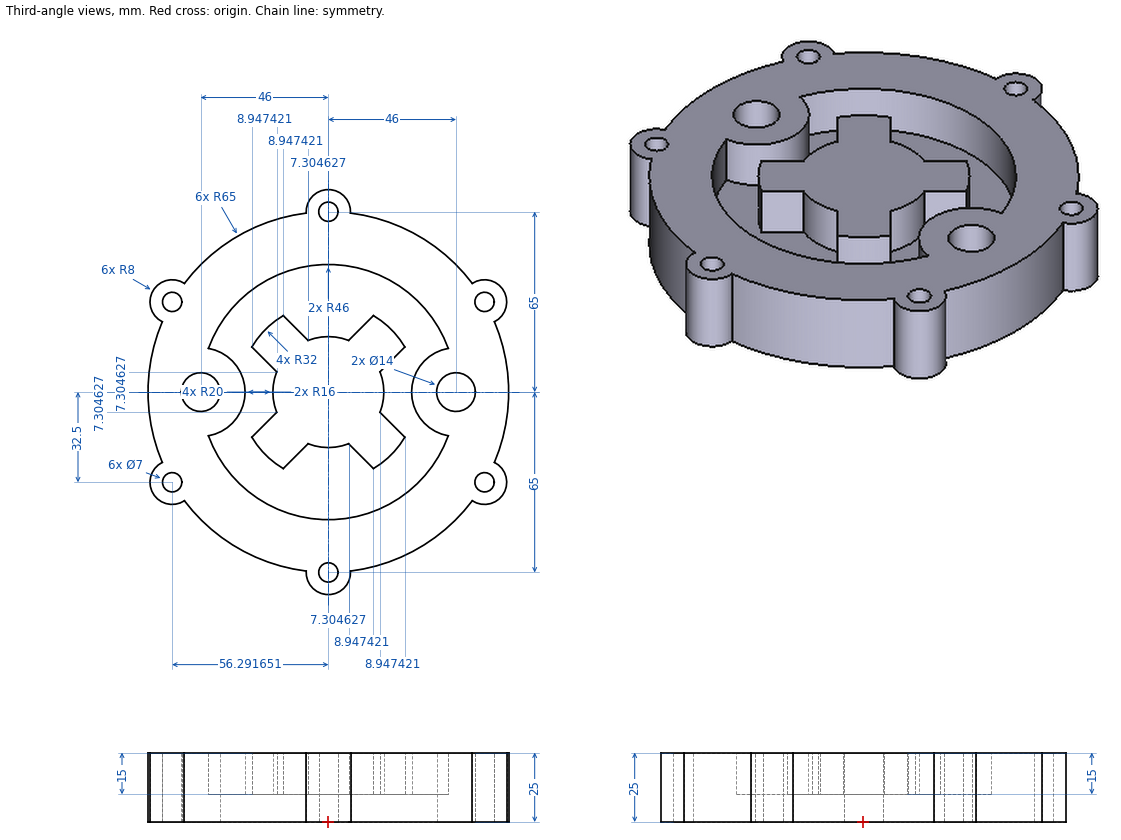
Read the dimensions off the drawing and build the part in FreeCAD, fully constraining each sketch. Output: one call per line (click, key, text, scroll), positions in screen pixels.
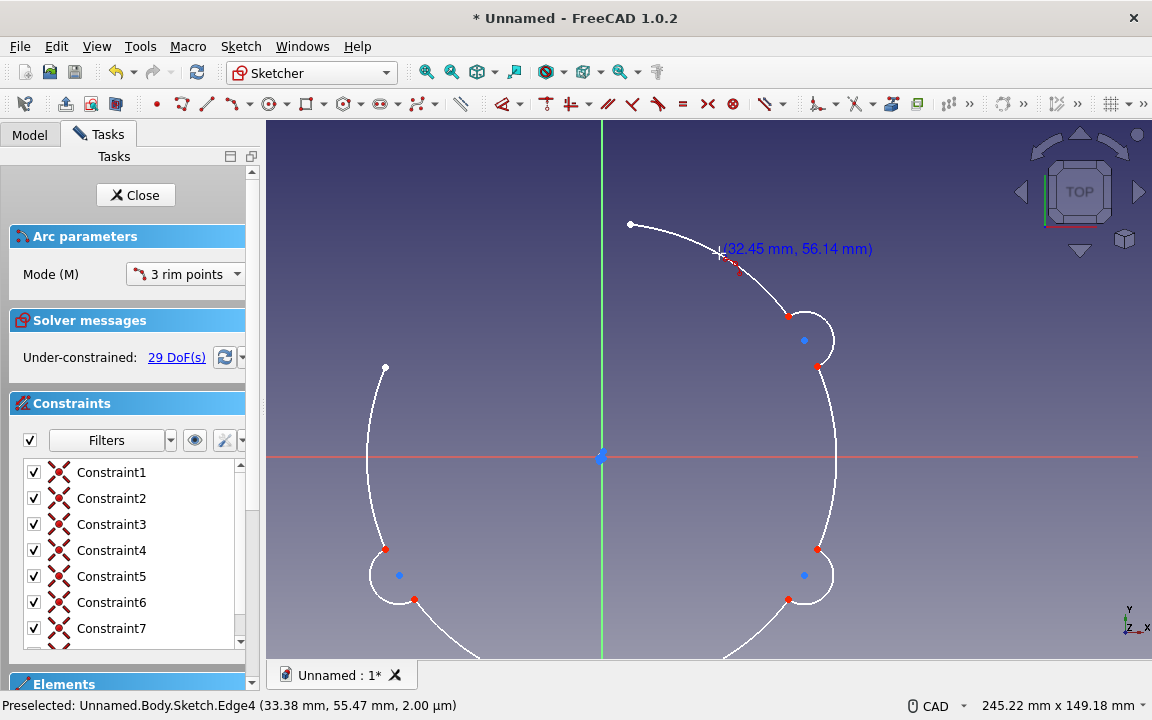
click(631, 225)
click(573, 224)
click(619, 199)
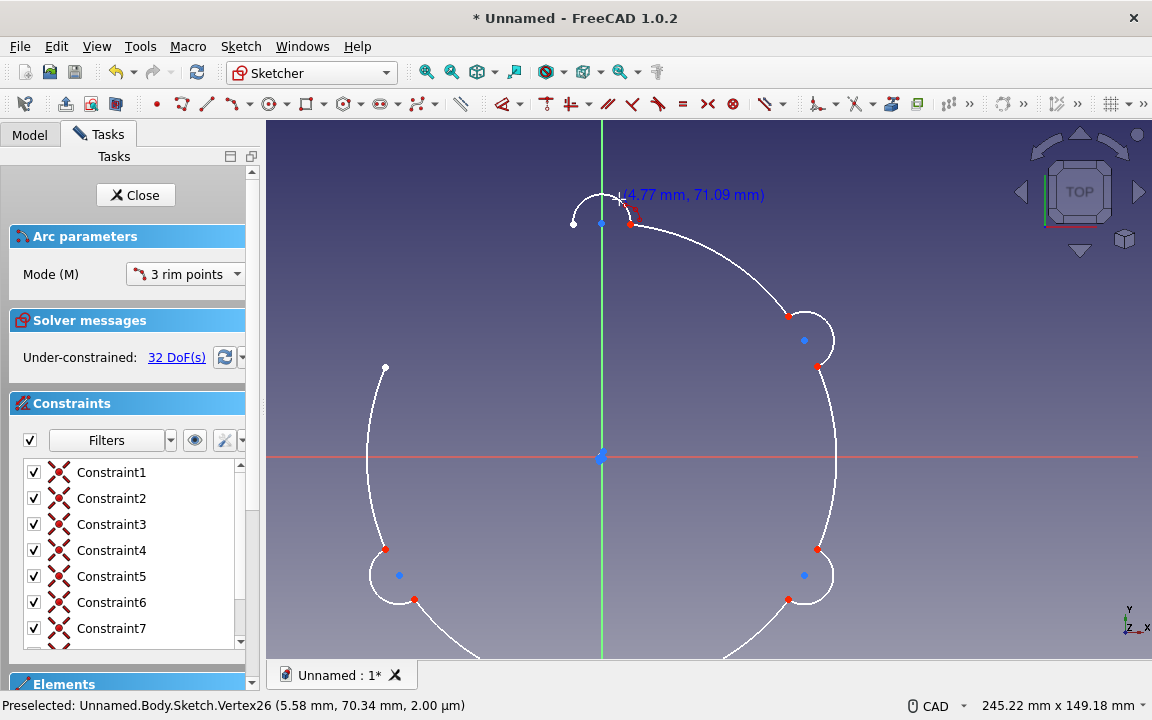
click(573, 225)
click(414, 315)
click(484, 253)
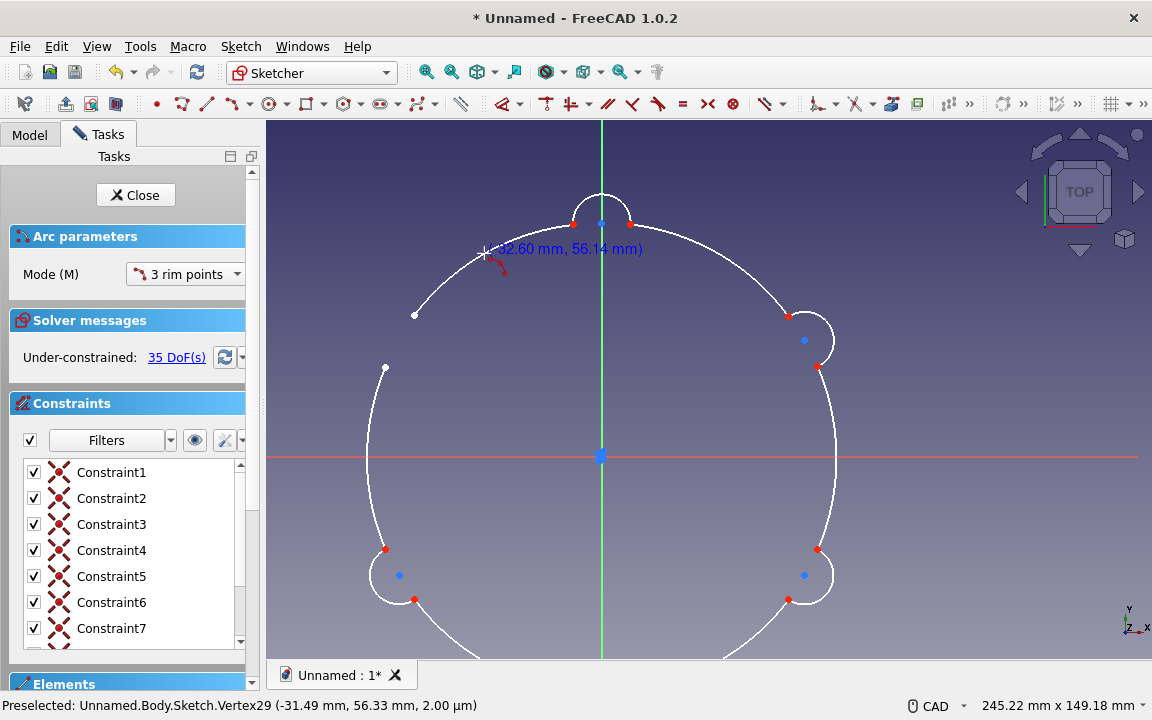
click(414, 316)
click(386, 367)
click(373, 325)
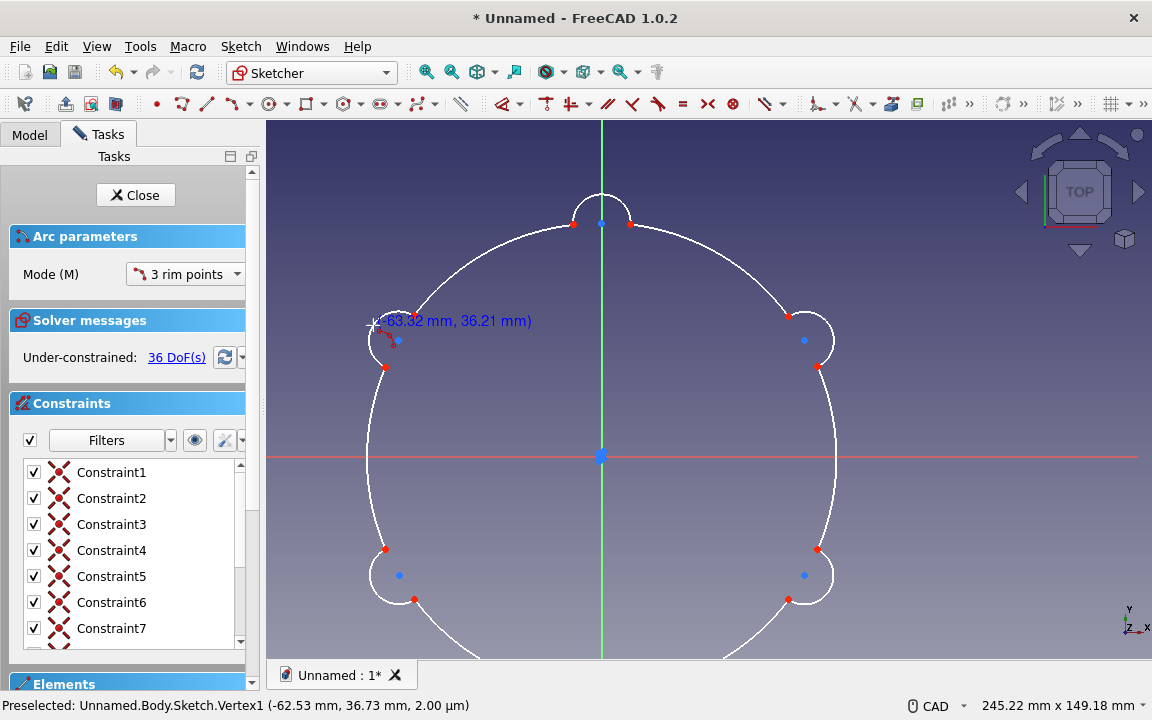
click(268, 104)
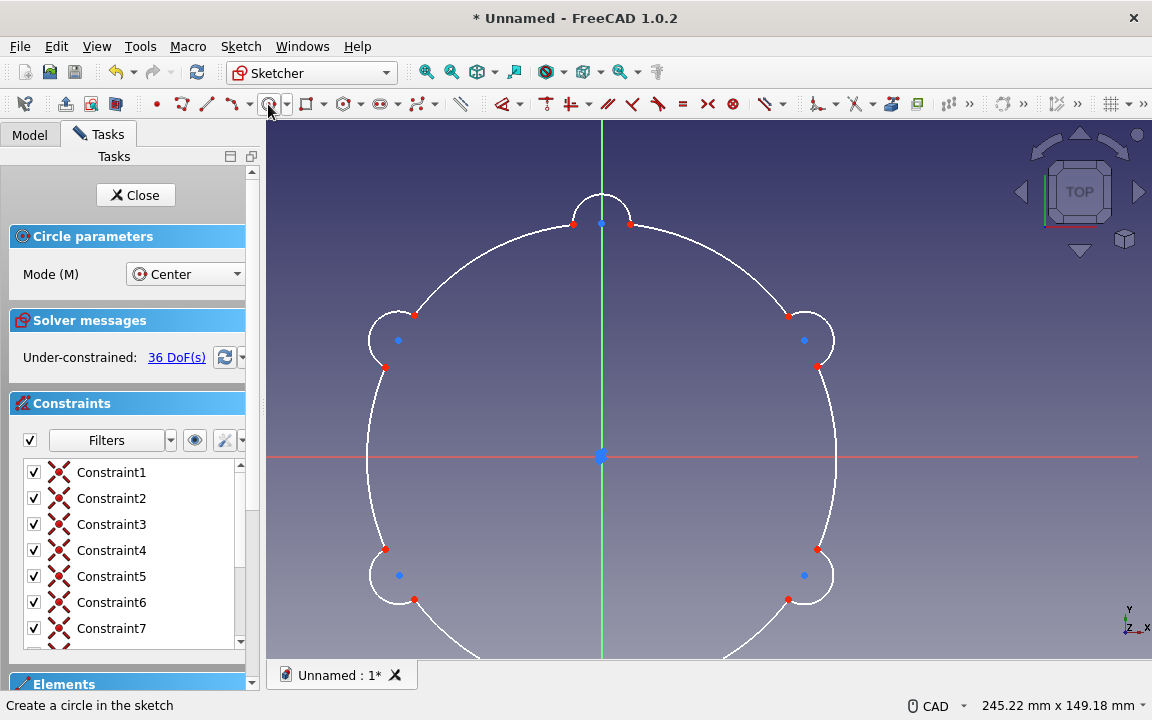
scroll(398, 574, up, 3)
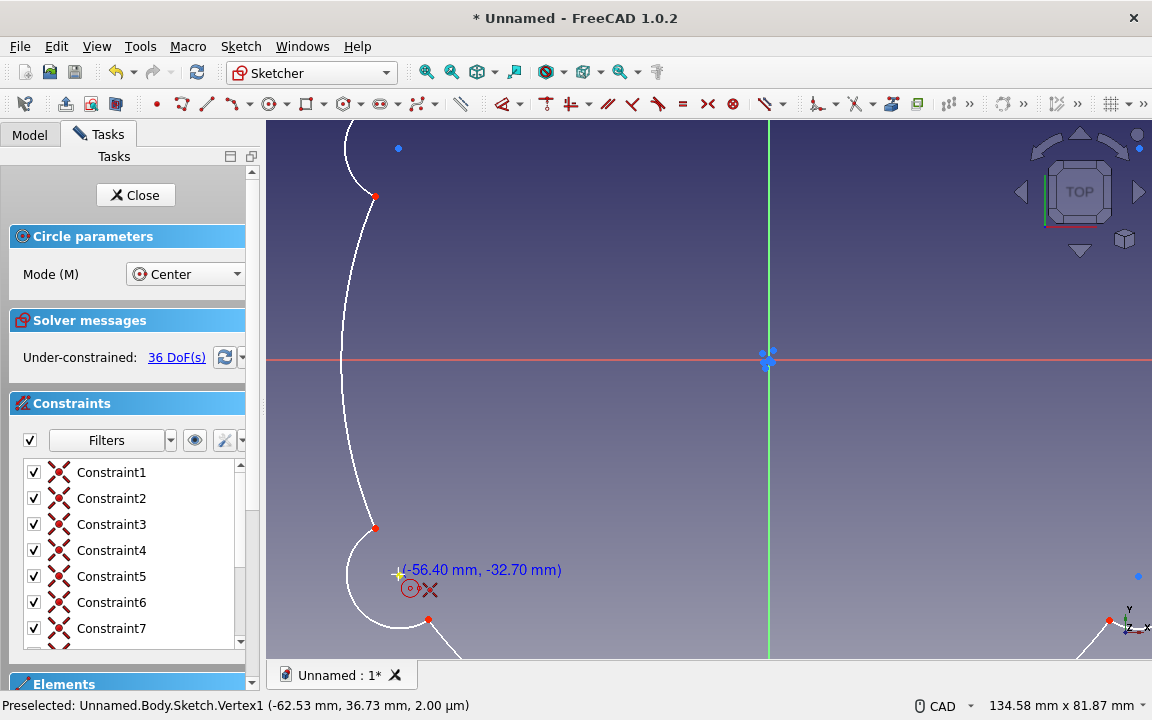
click(399, 574)
click(415, 557)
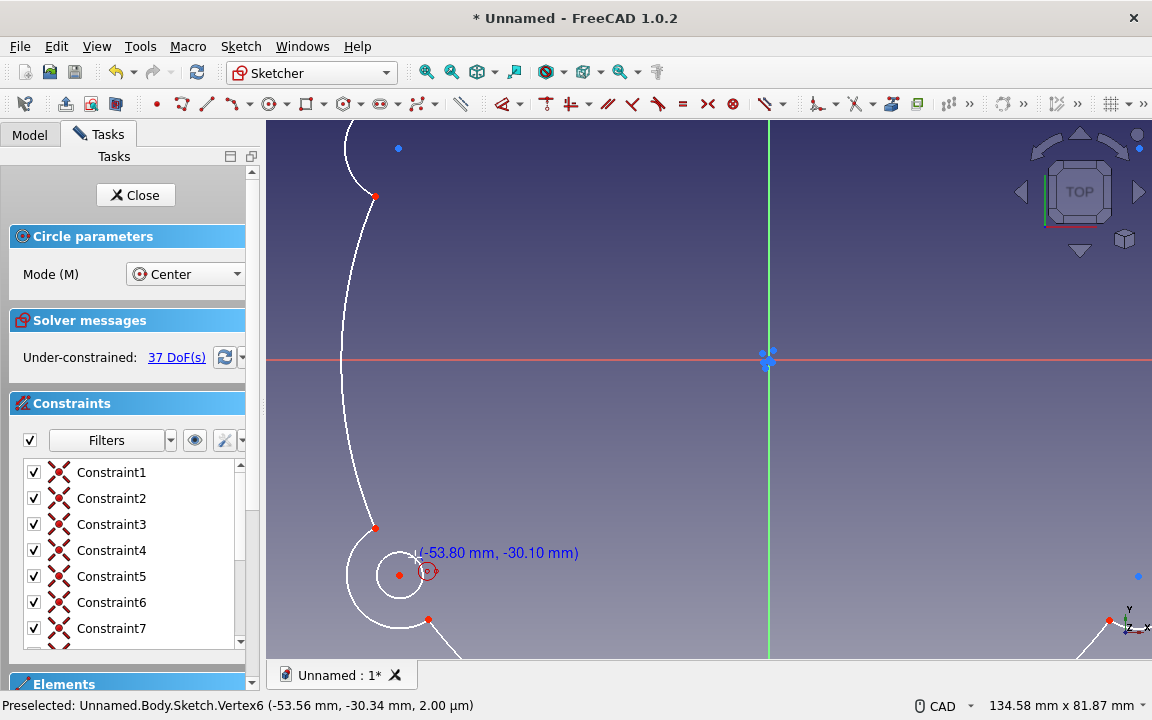
scroll(566, 407, down, 5)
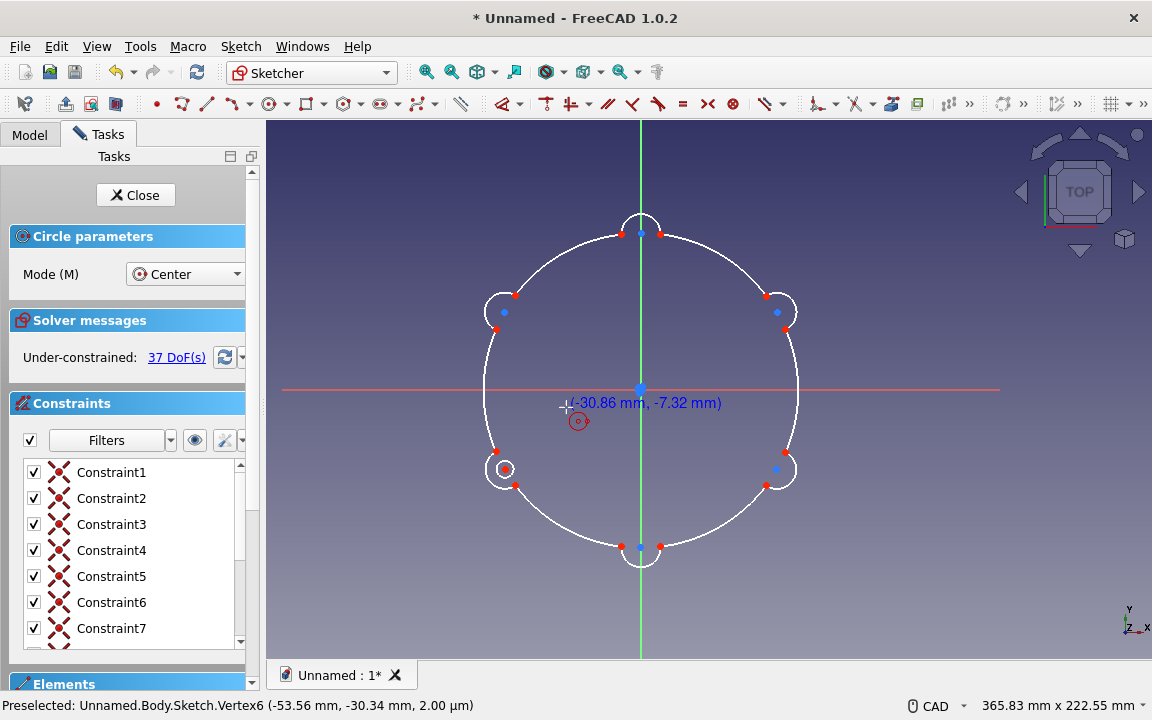
scroll(641, 547, up, 5)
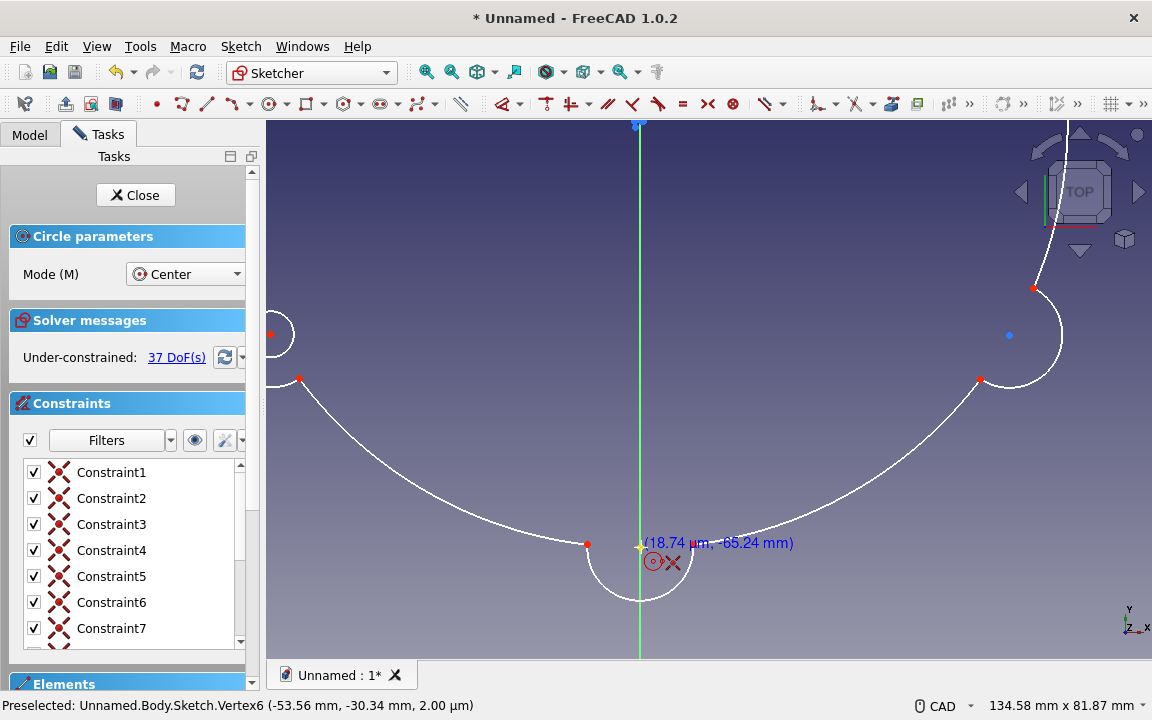
click(640, 547)
click(656, 530)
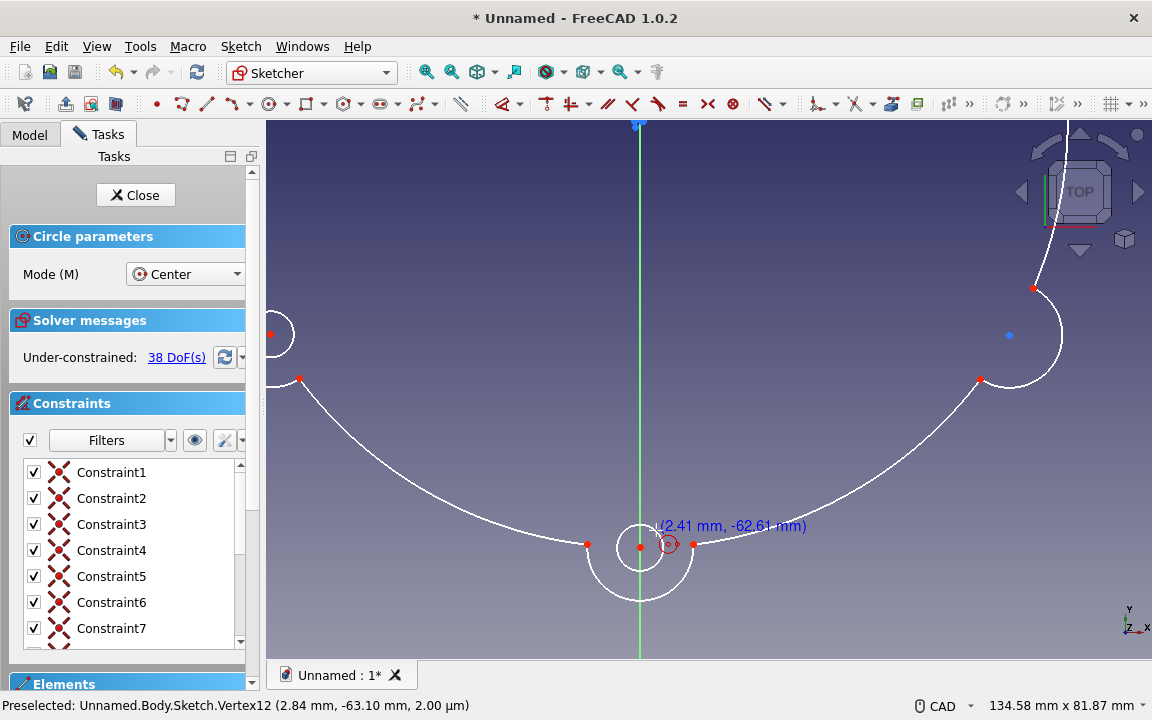
scroll(641, 547, down, 5)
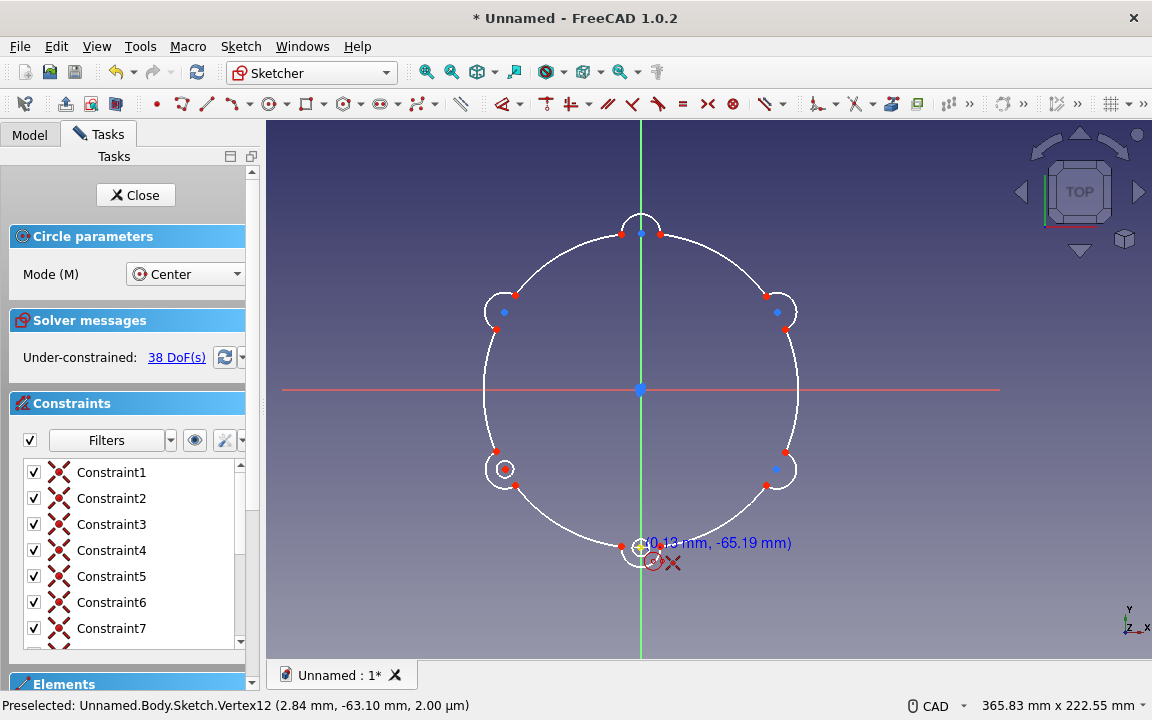
scroll(777, 469, up, 5)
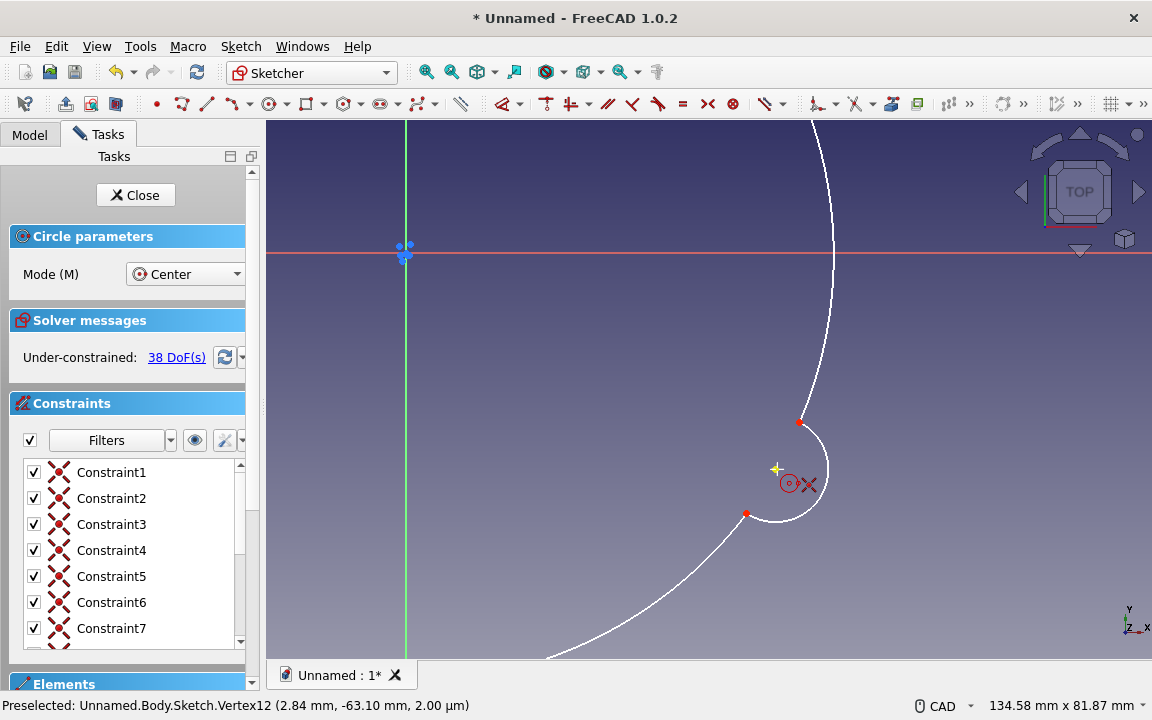
click(777, 467)
click(793, 451)